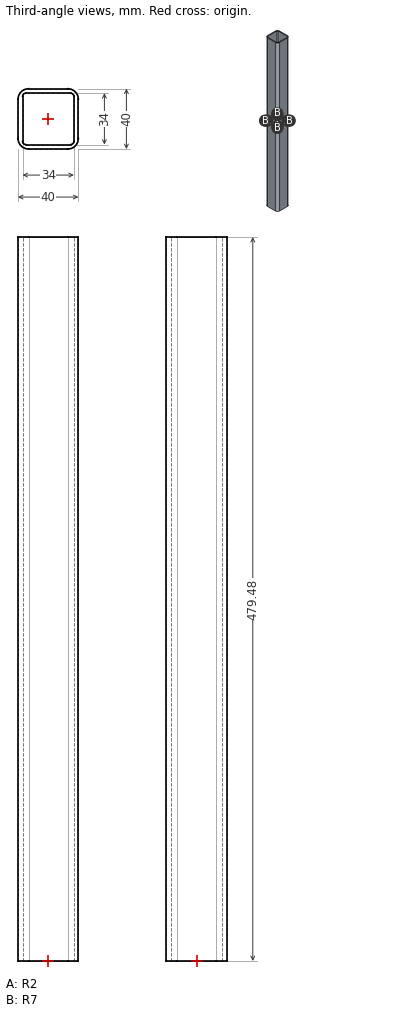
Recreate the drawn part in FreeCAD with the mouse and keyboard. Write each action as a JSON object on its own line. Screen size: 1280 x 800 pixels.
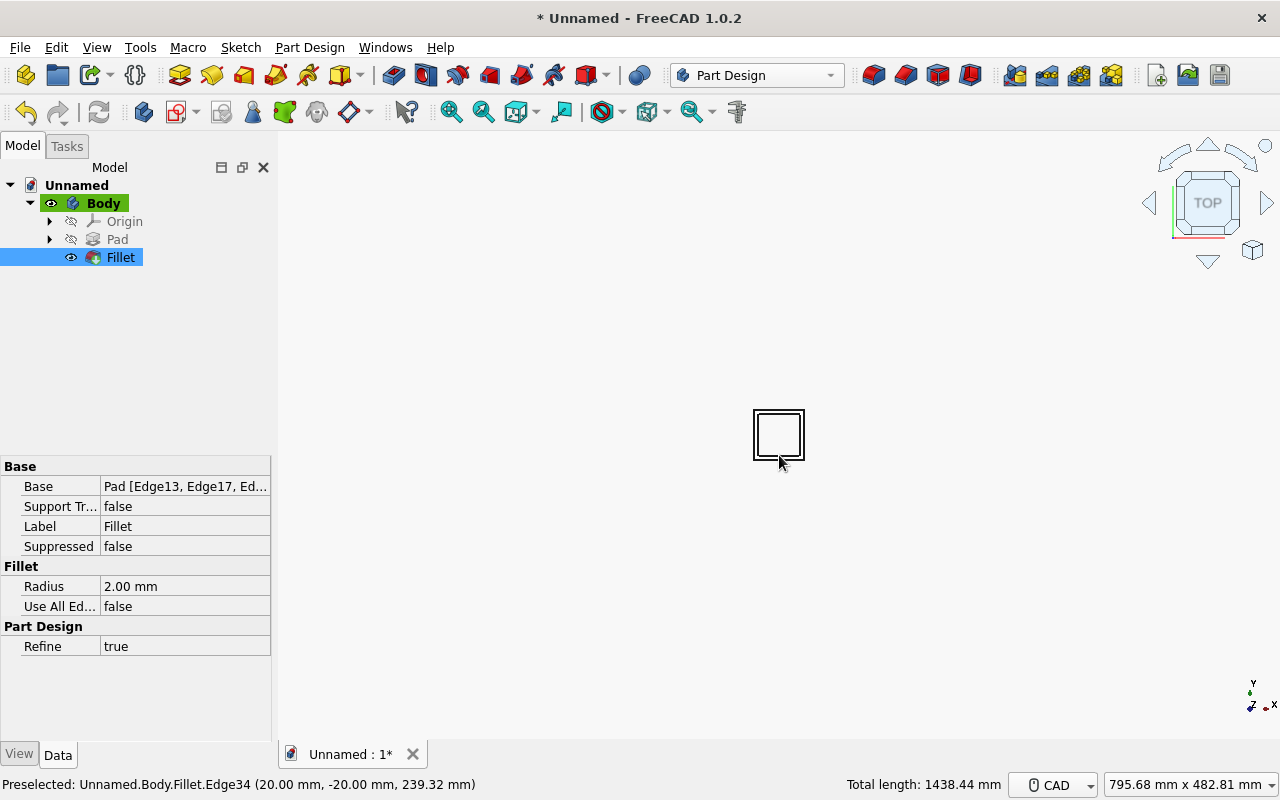
{"action": "key", "text": "v f"}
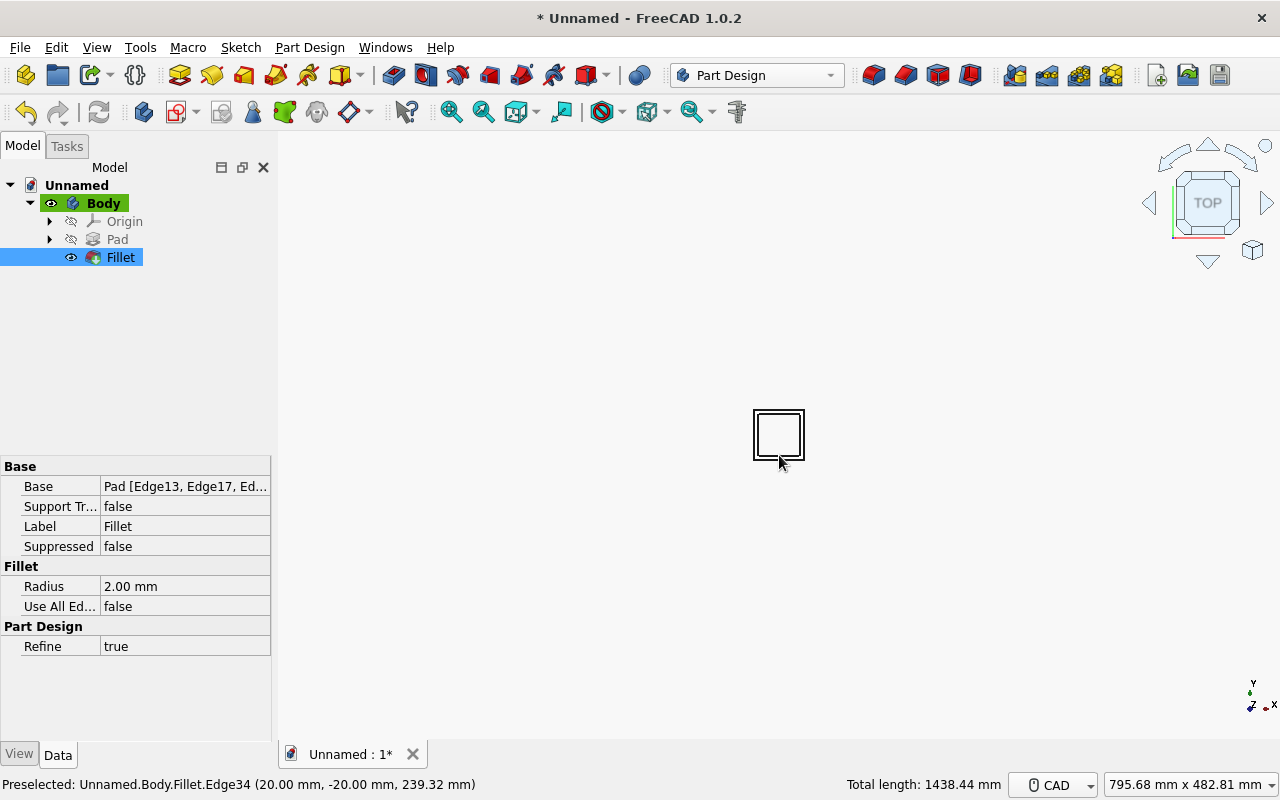
{"action": "key", "text": "1"}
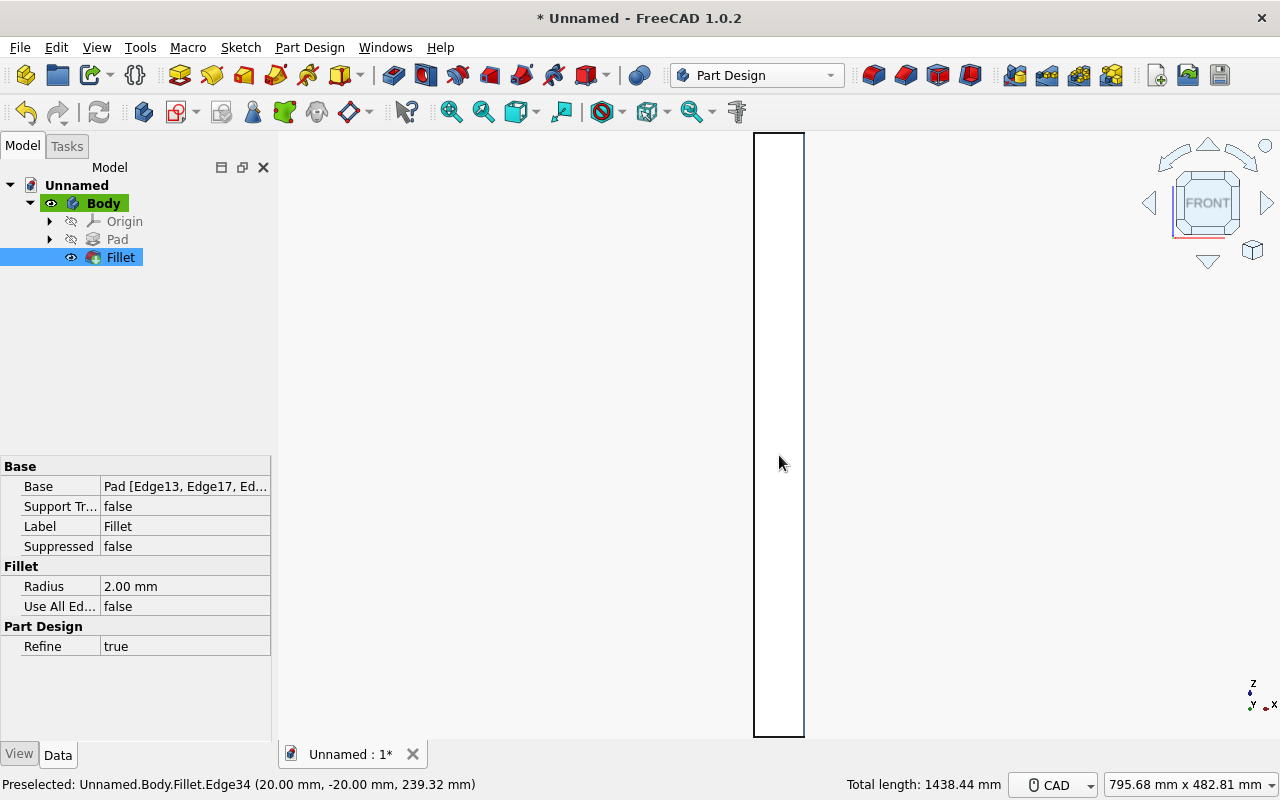
{"action": "left_click", "coordinate": [754, 434], "text": "ctrl"}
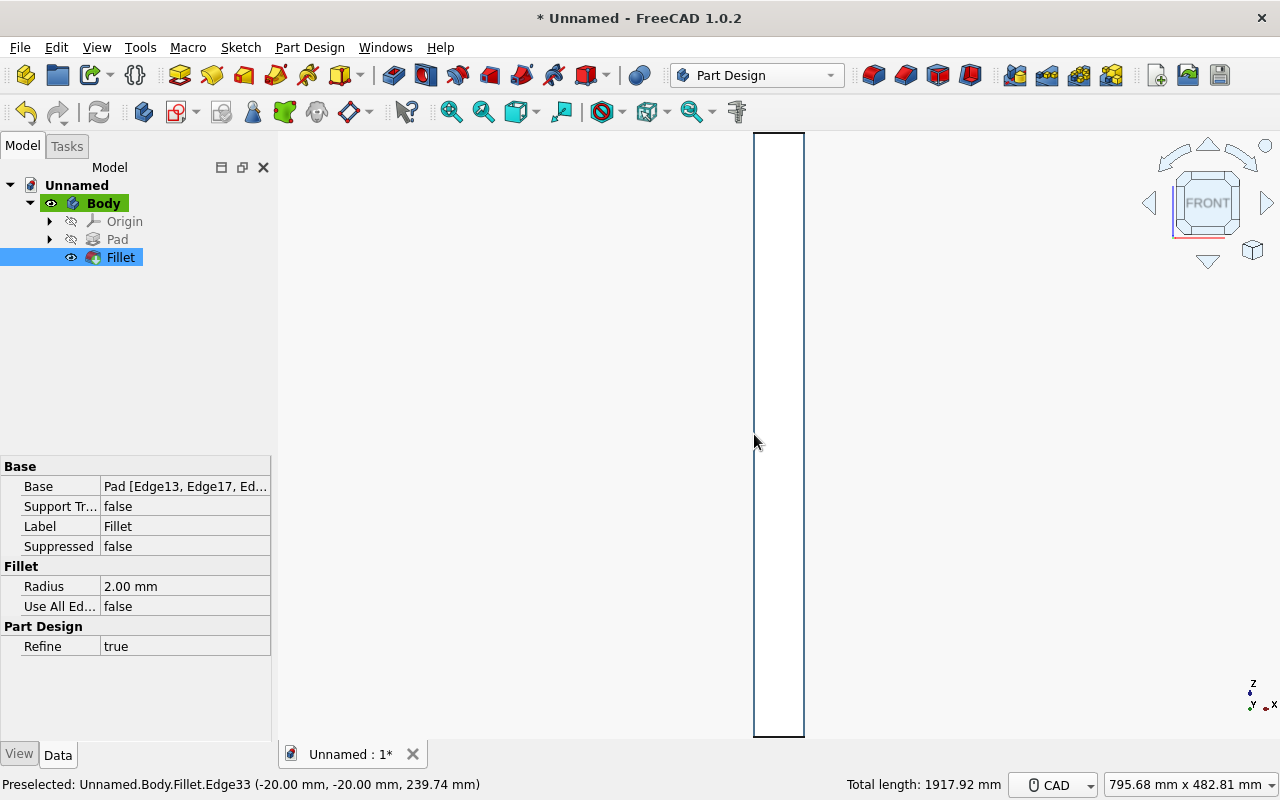
{"action": "left_click", "coordinate": [874, 76]}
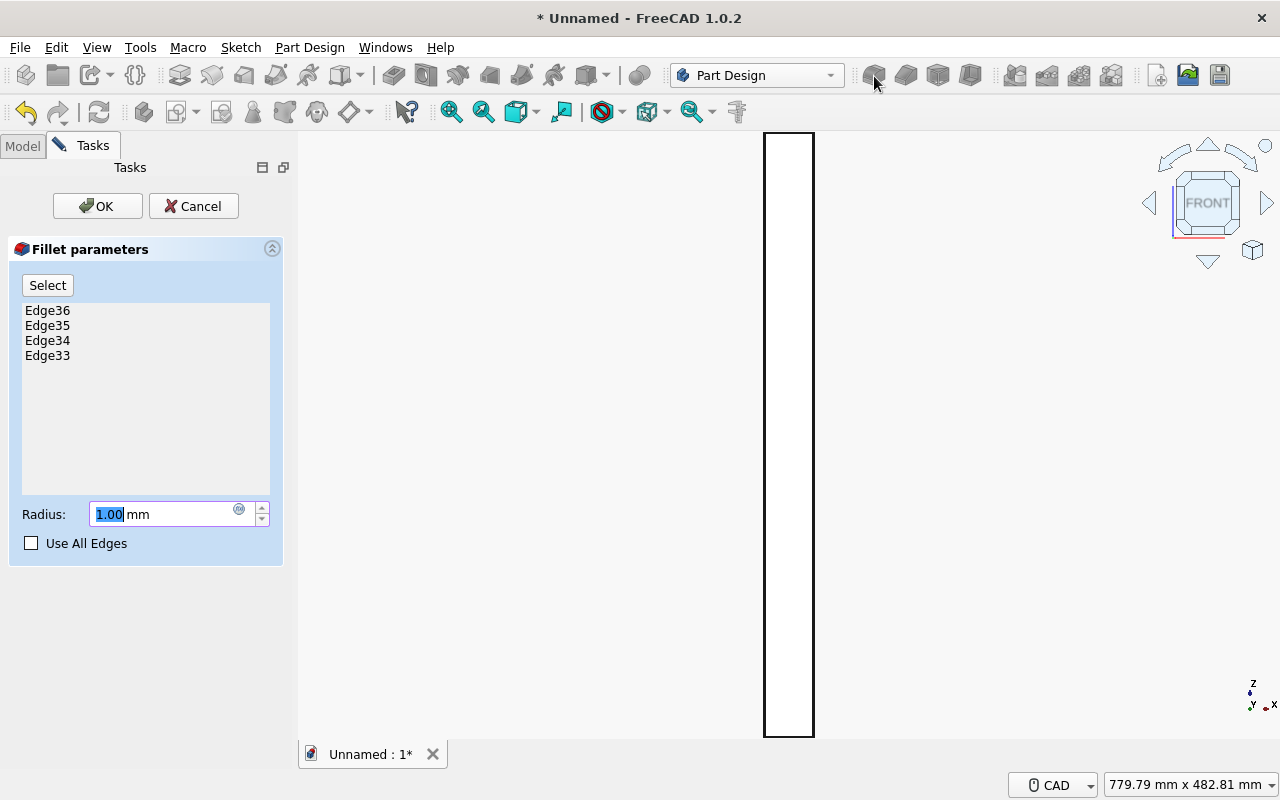
{"action": "type", "text": "7"}
{"action": "key", "text": "Tab"}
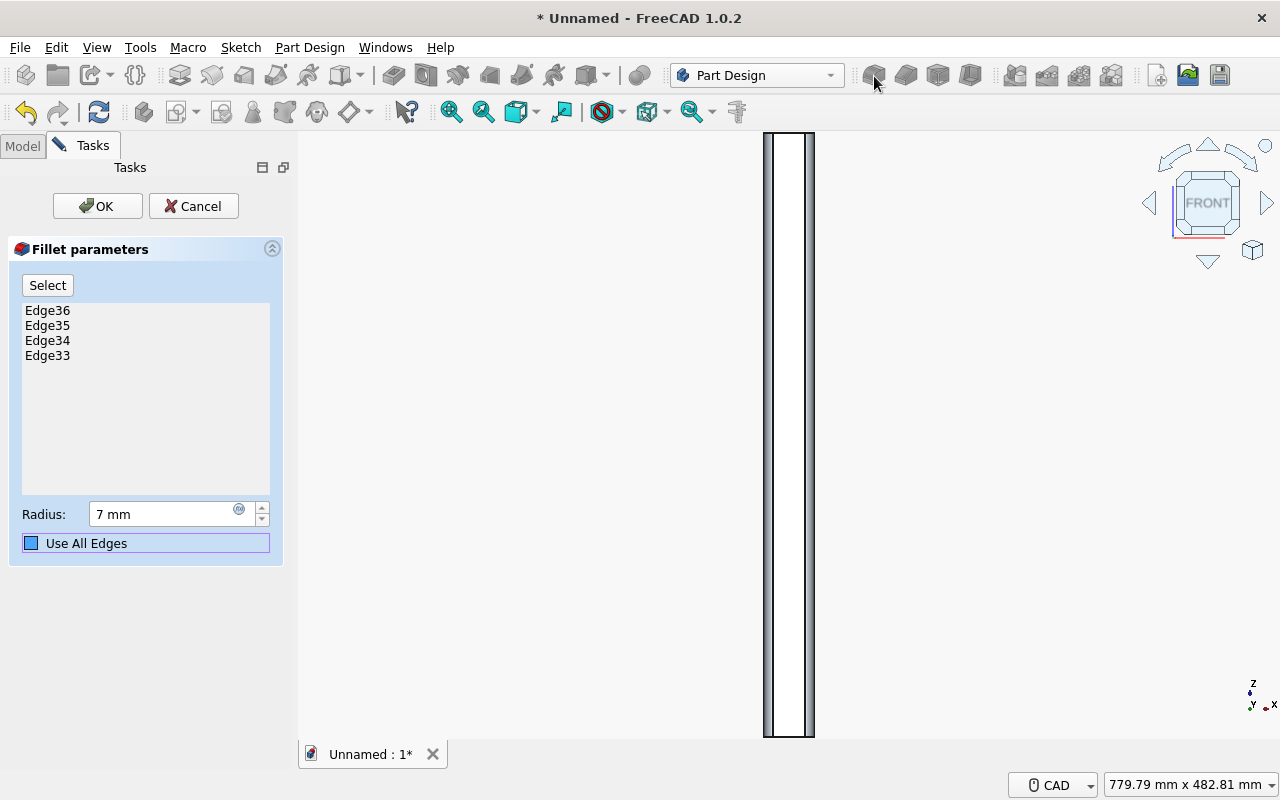
{"action": "left_click", "coordinate": [98, 206]}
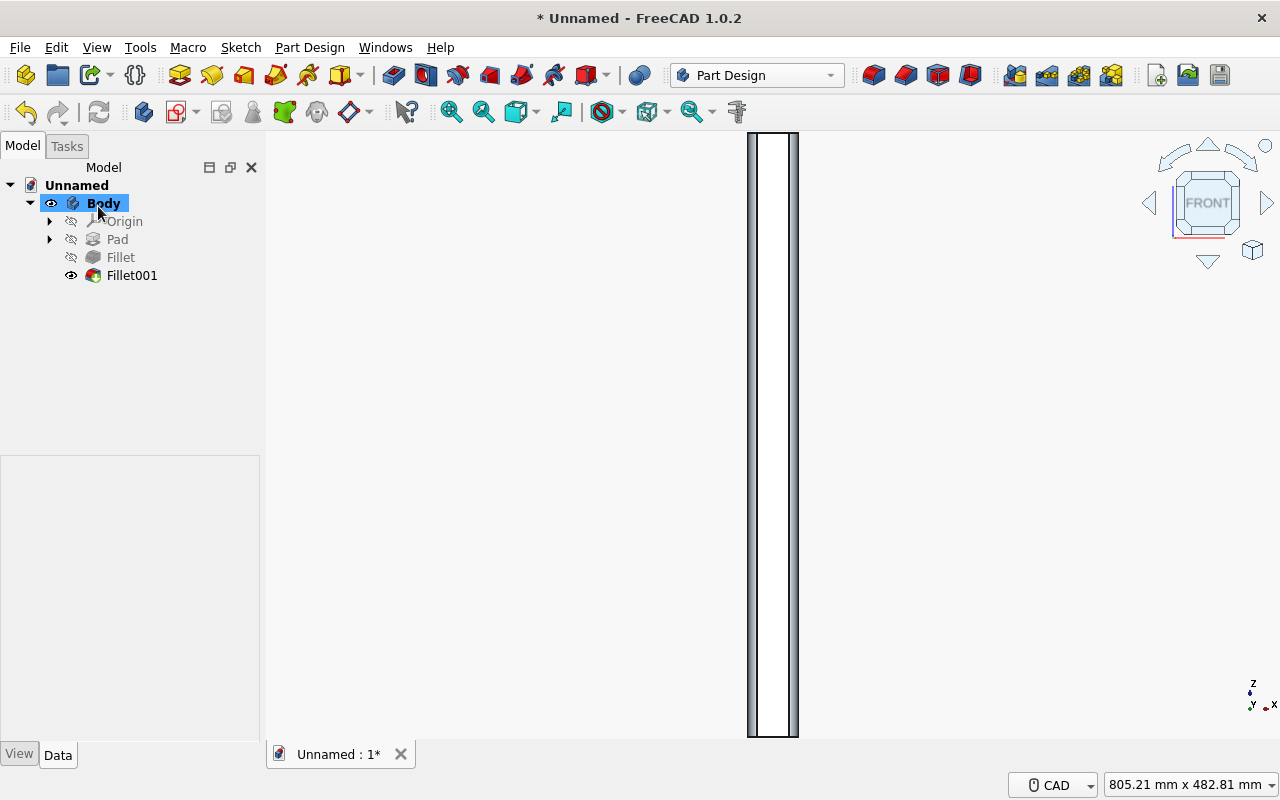
{"action": "key", "text": "0"}